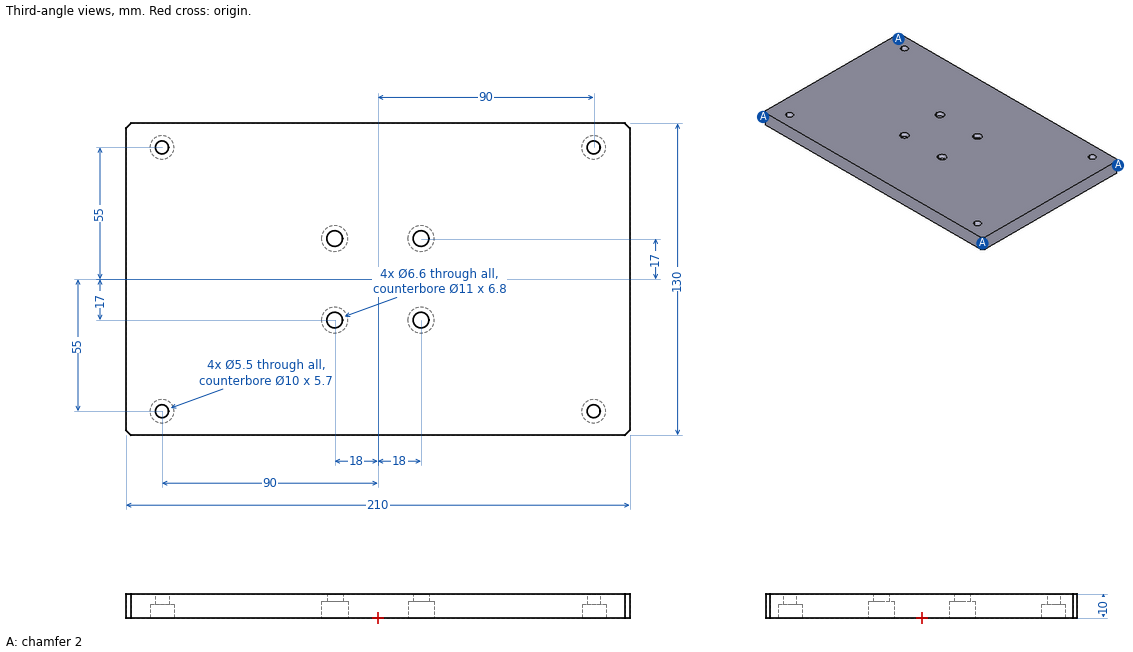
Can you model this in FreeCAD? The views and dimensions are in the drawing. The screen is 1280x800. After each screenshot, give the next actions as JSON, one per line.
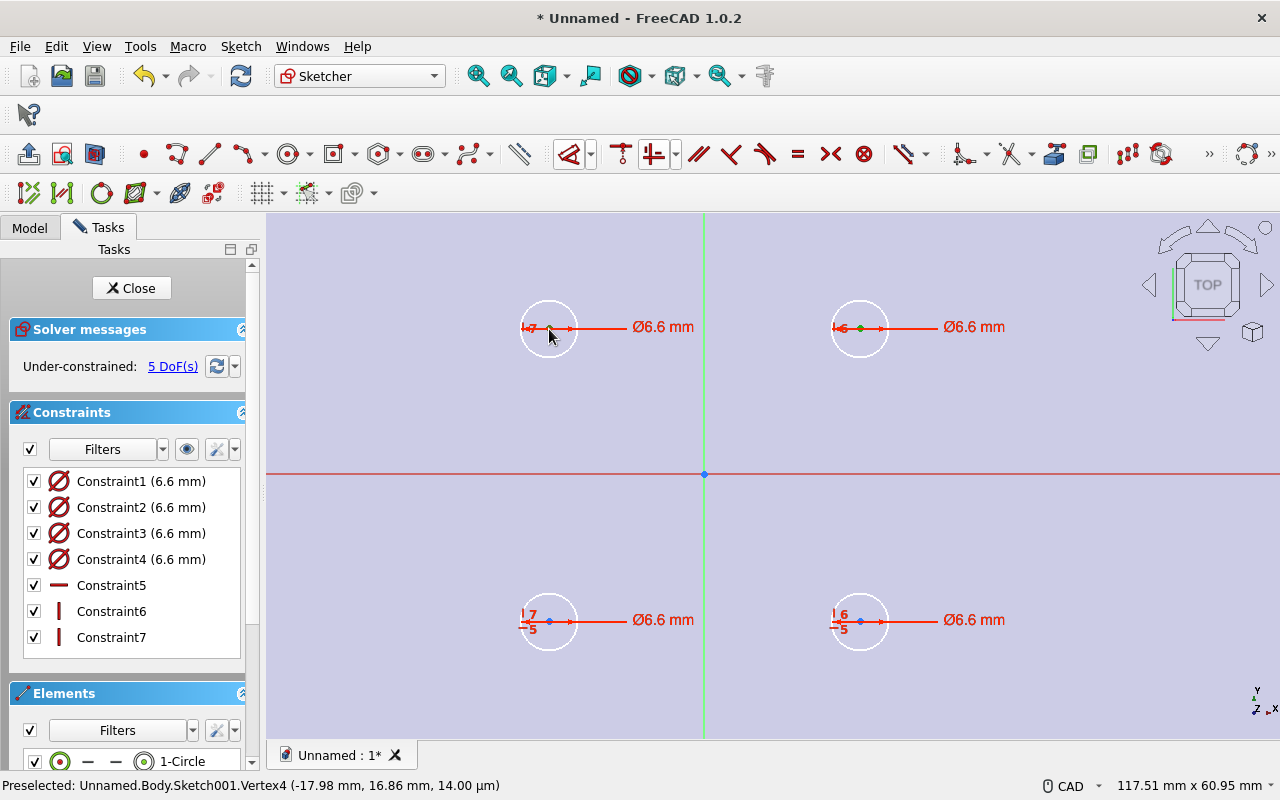
{"action": "key", "text": "h"}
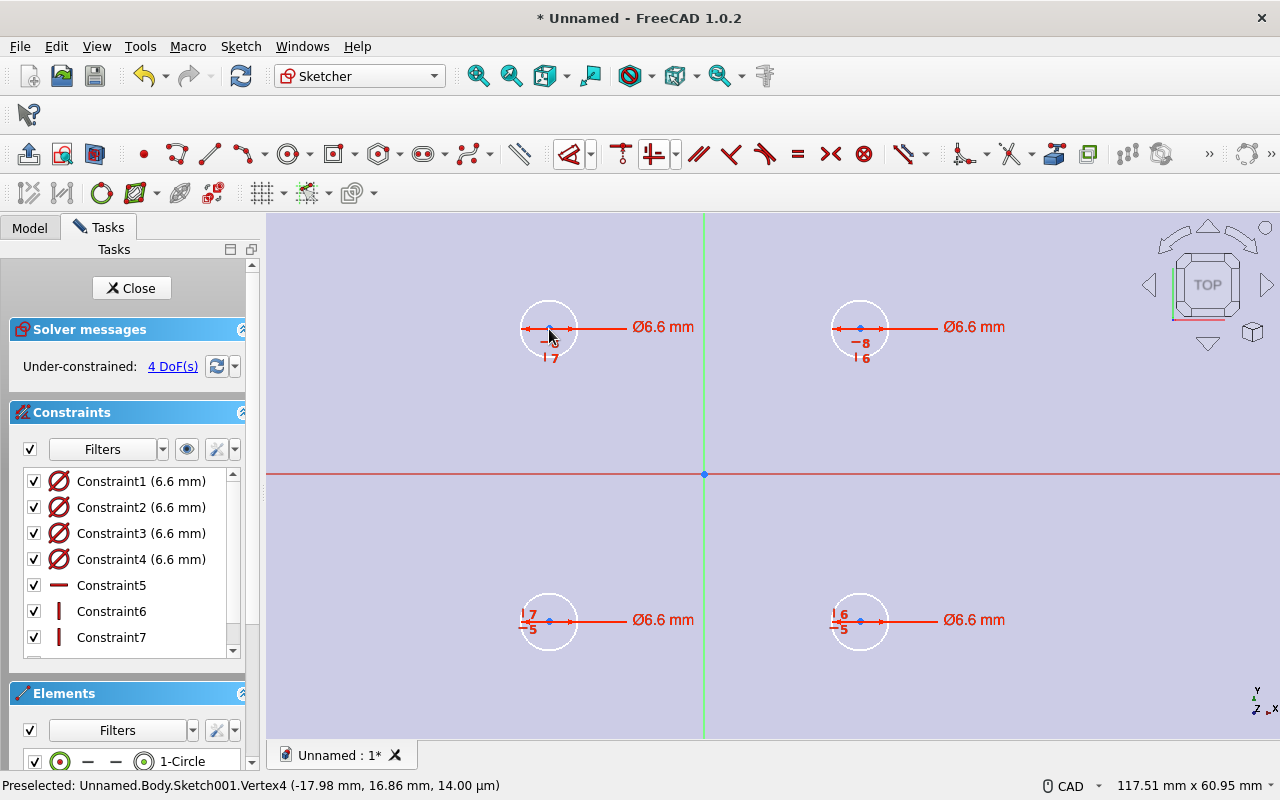
{"action": "key", "text": "d"}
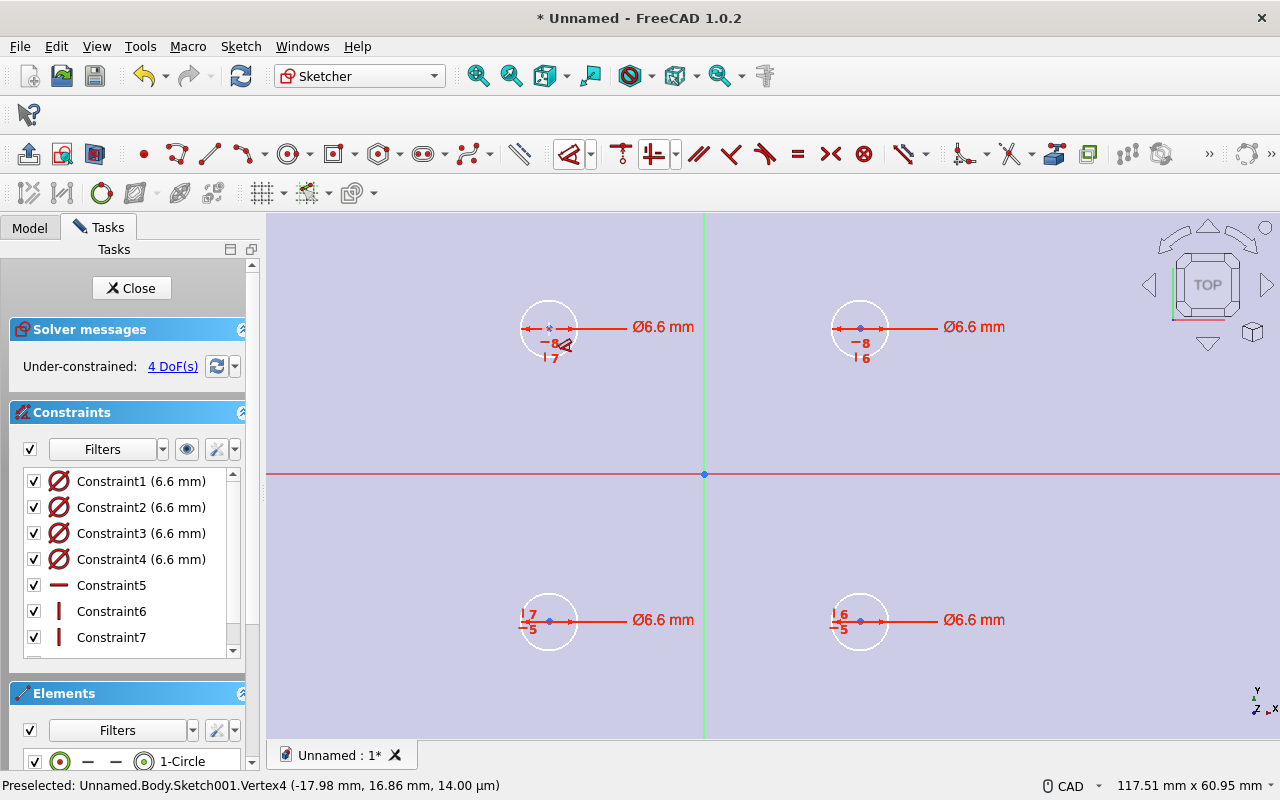
{"action": "left_click", "coordinate": [549, 622]}
{"action": "left_click", "coordinate": [627, 656]}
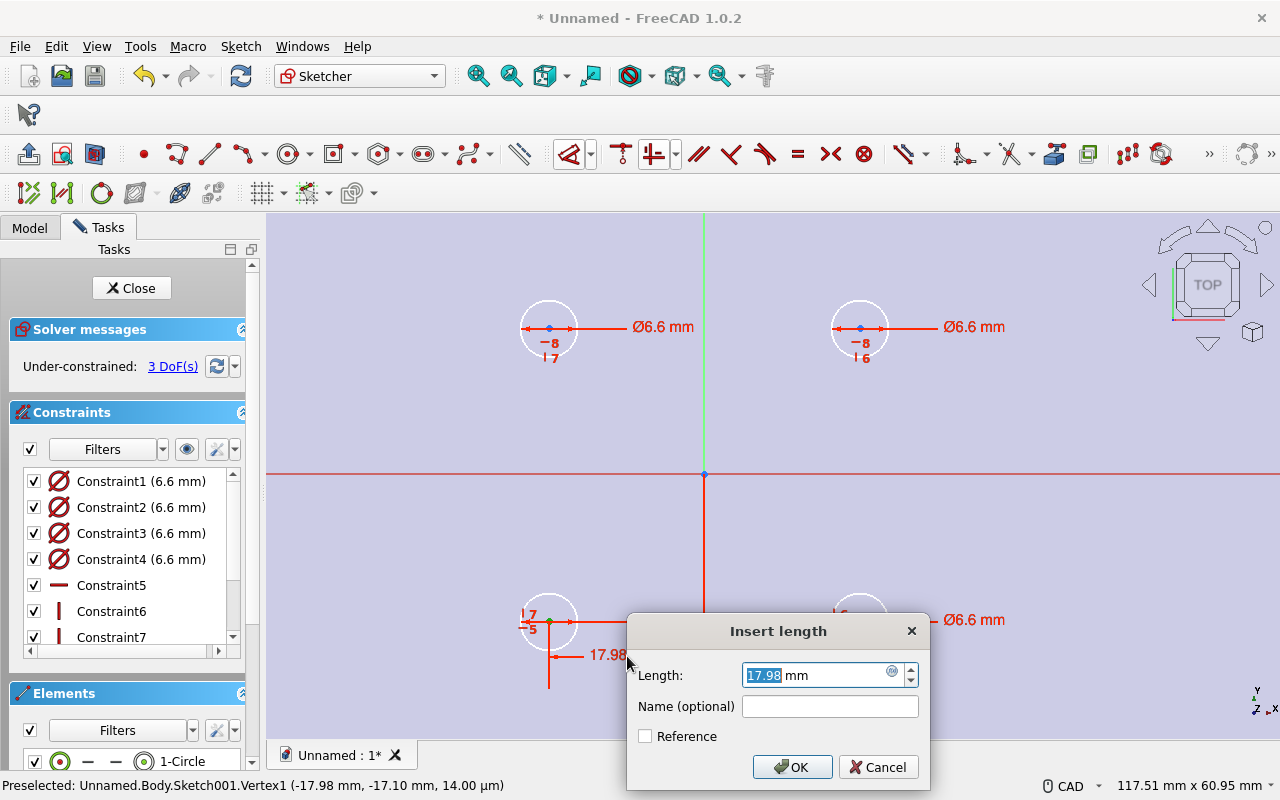
{"action": "type", "text": "18"}
{"action": "key", "text": "Return"}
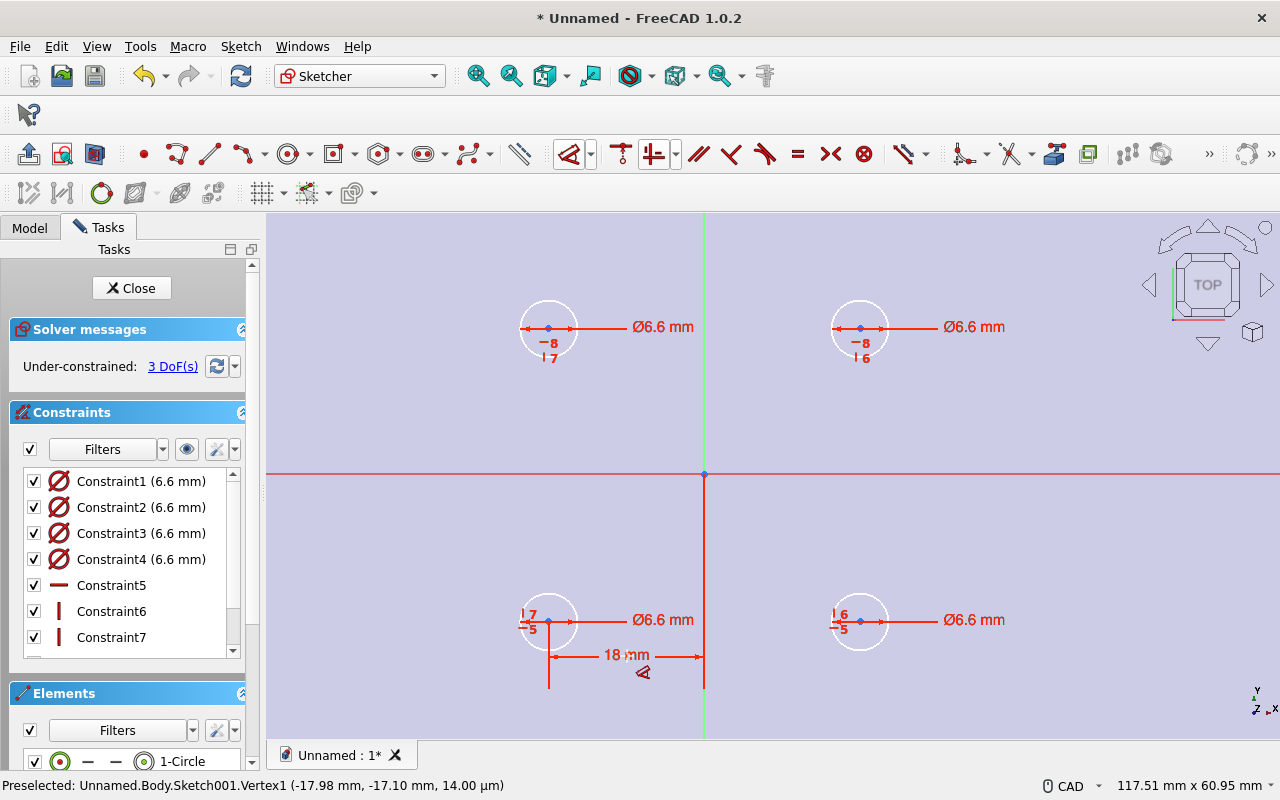
{"action": "left_click", "coordinate": [549, 622]}
{"action": "left_click", "coordinate": [515, 548]}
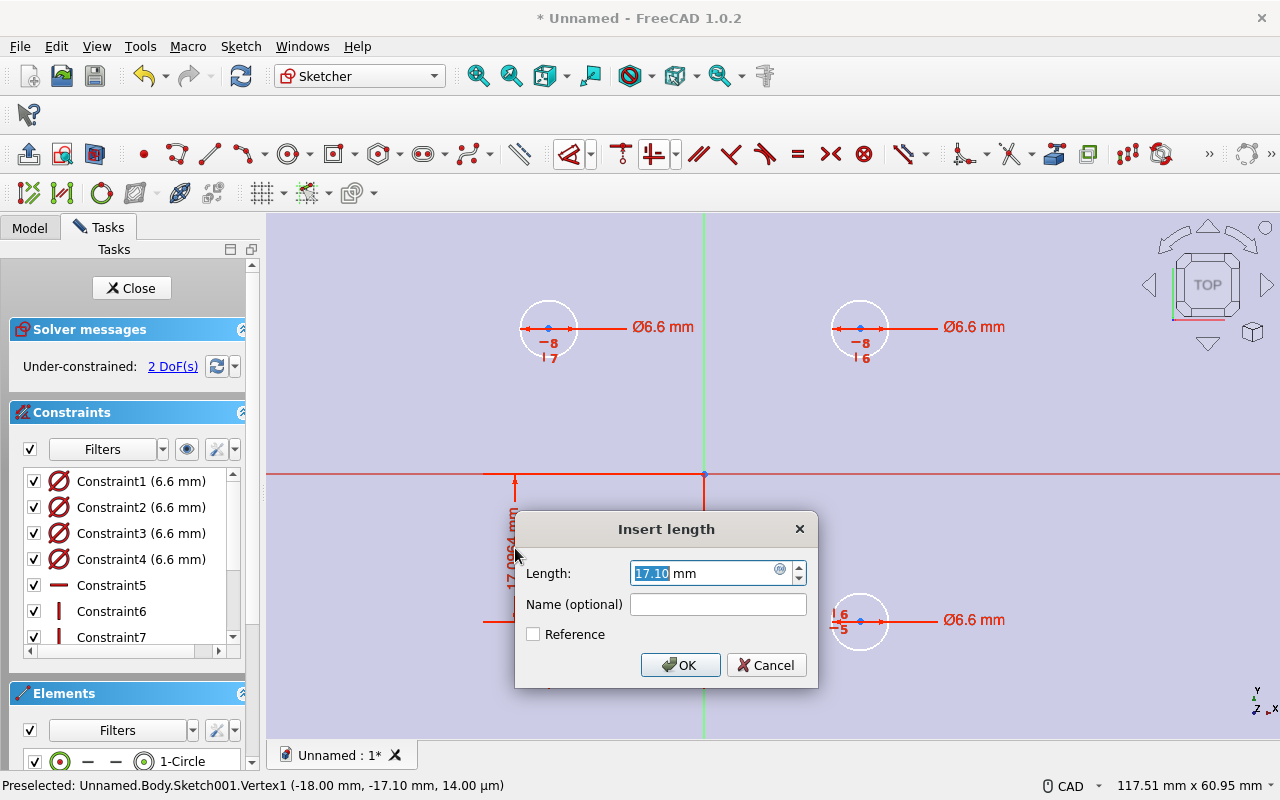
{"action": "type", "text": "17"}
{"action": "key", "text": "Return"}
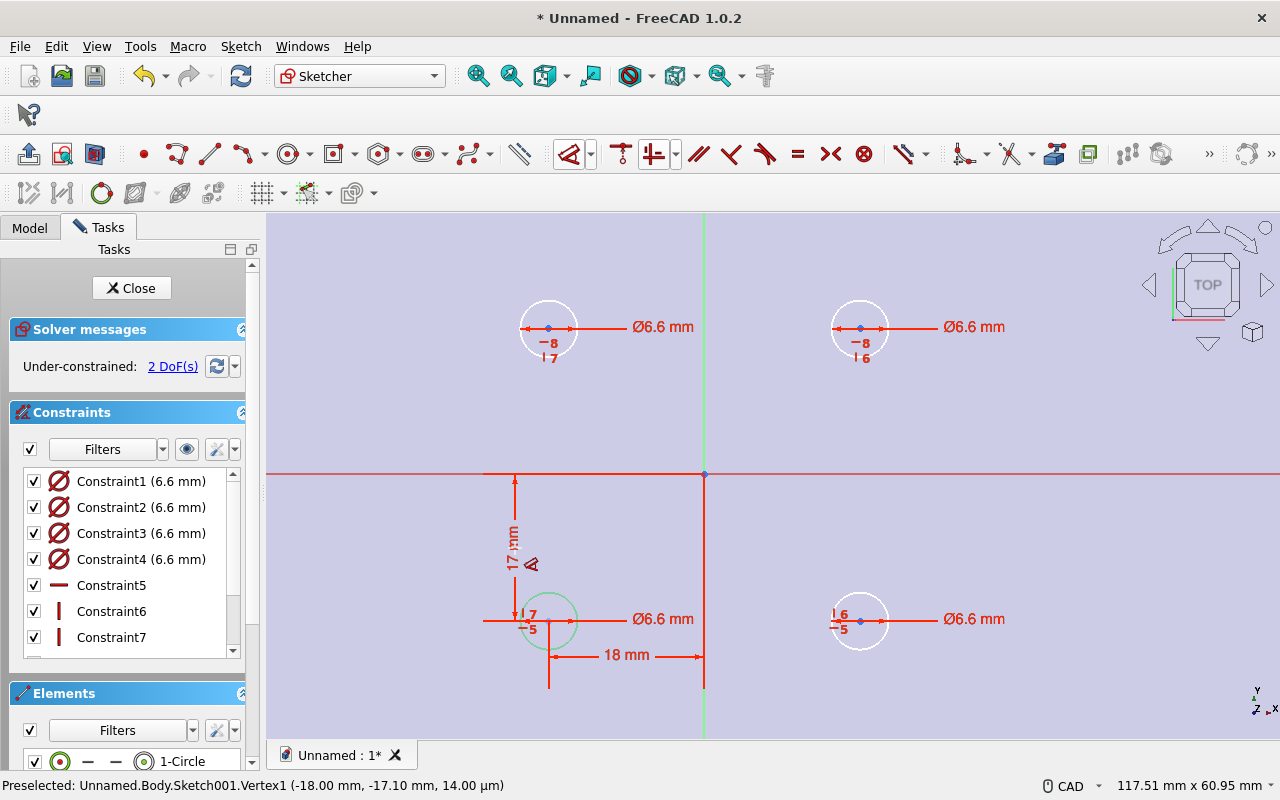
{"action": "left_click", "coordinate": [860, 621]}
{"action": "left_click", "coordinate": [782, 655]}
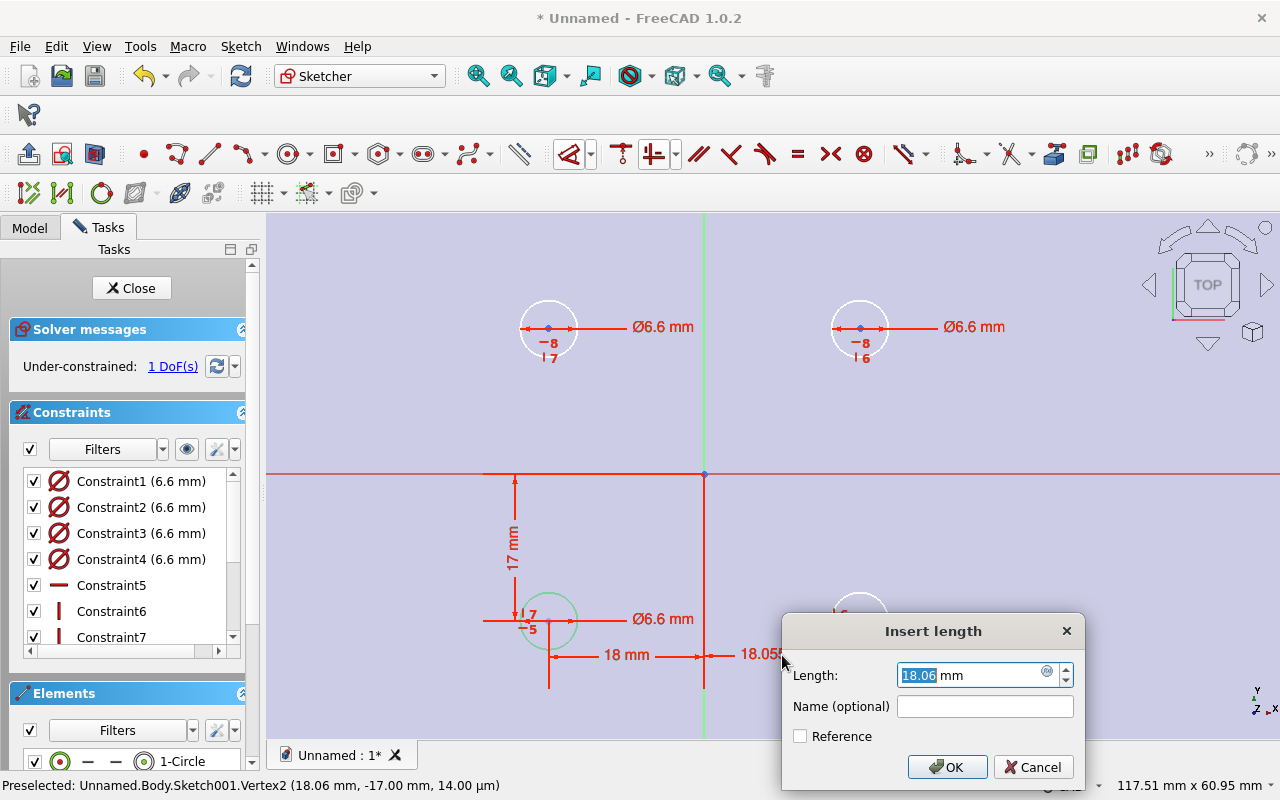
{"action": "type", "text": "18"}
{"action": "key", "text": "Return"}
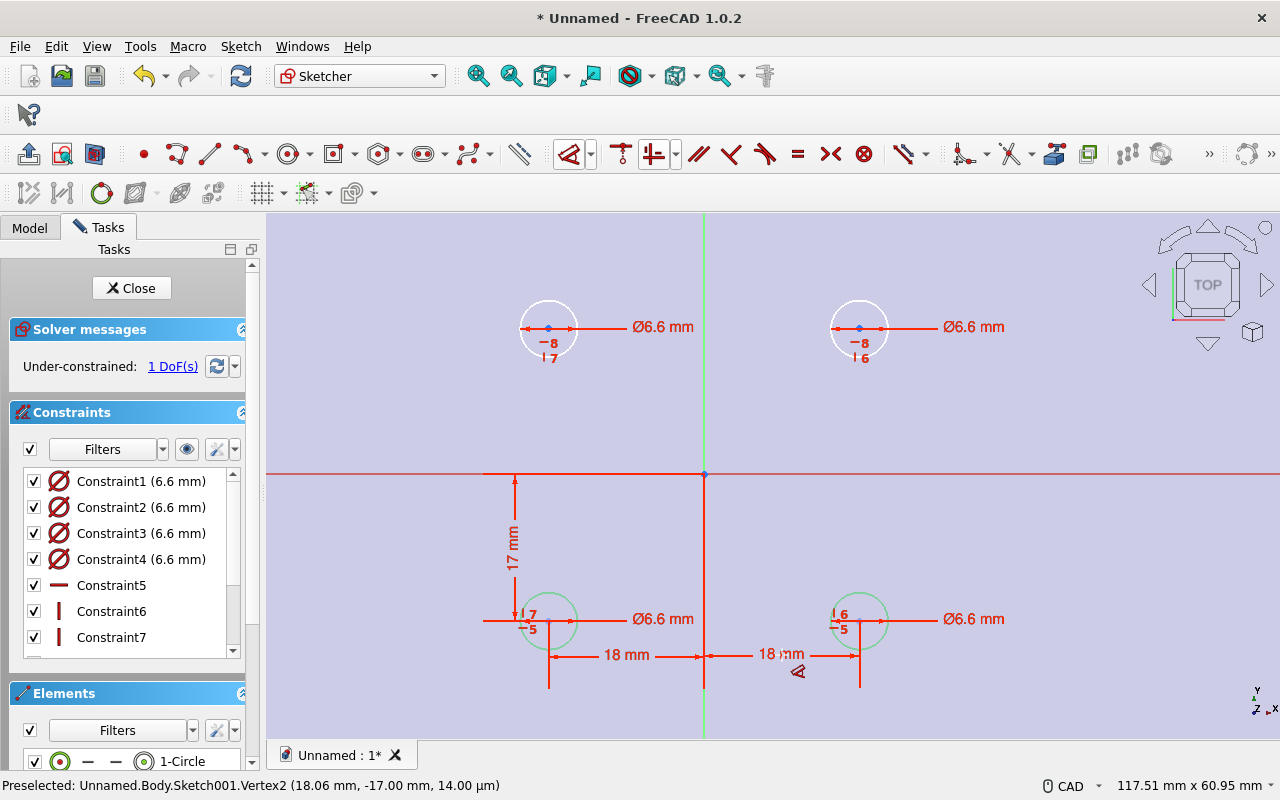
{"action": "left_click", "coordinate": [860, 329]}
{"action": "left_click", "coordinate": [894, 402]}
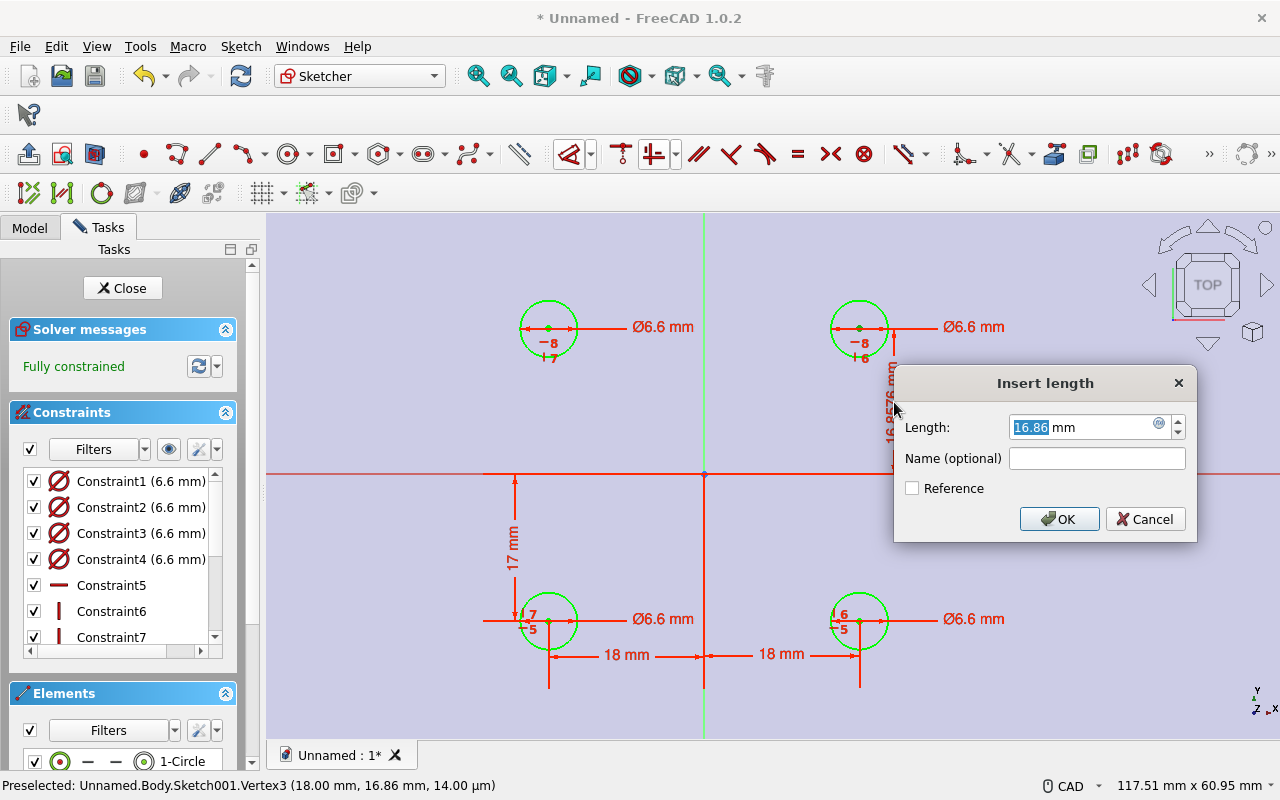
{"action": "type", "text": "17"}
{"action": "key", "text": "Return"}
{"action": "key", "text": "Escape"}